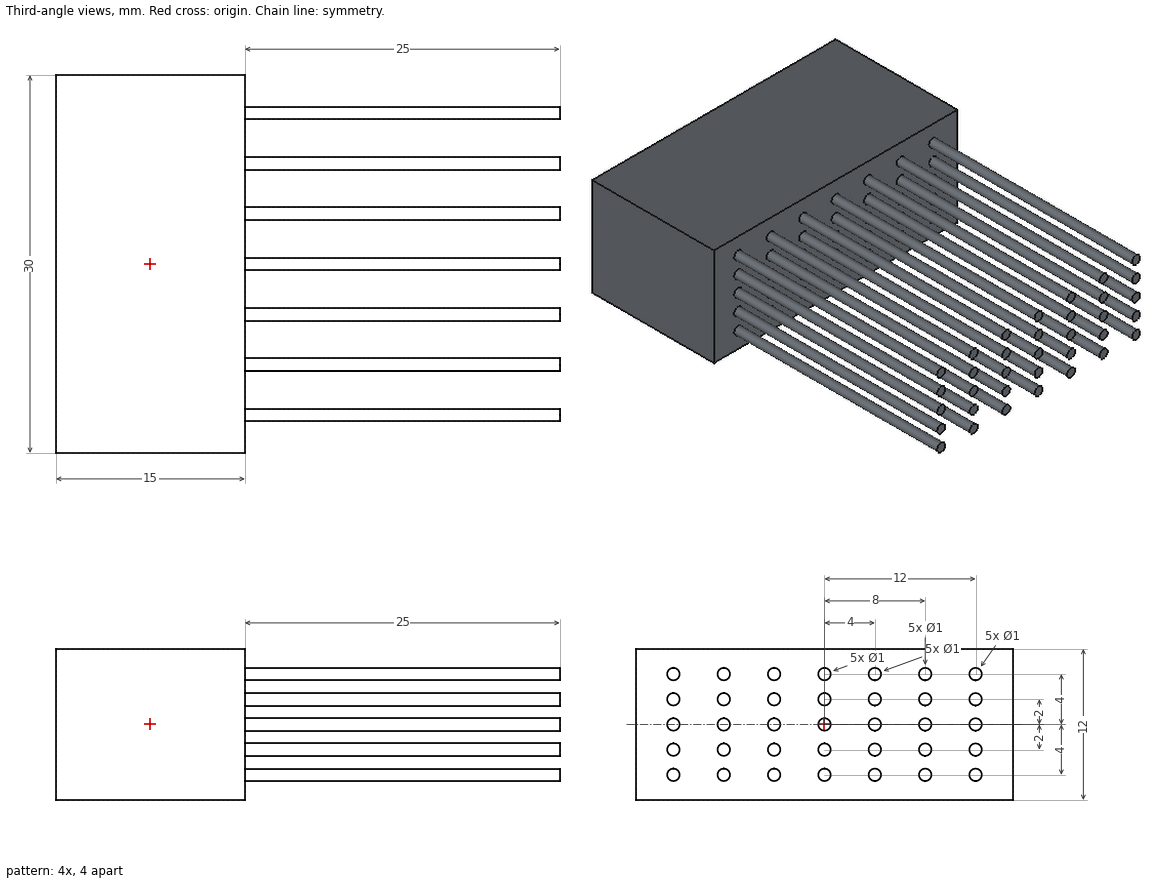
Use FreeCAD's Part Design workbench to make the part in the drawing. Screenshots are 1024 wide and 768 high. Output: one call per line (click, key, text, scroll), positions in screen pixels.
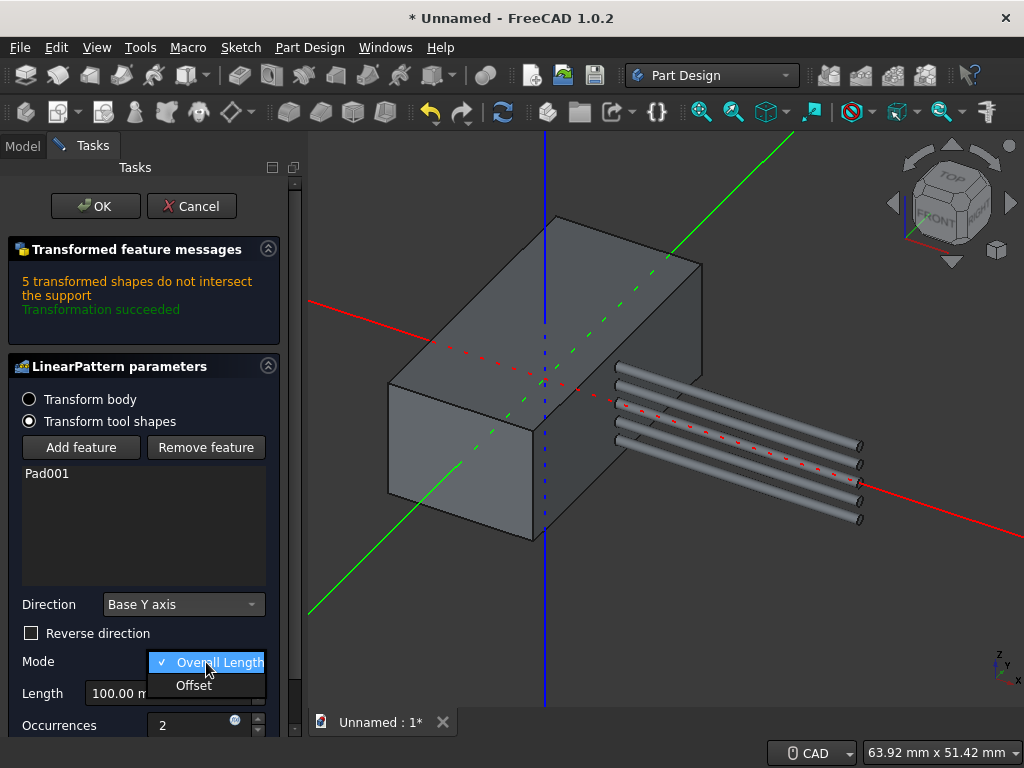
click(206, 686)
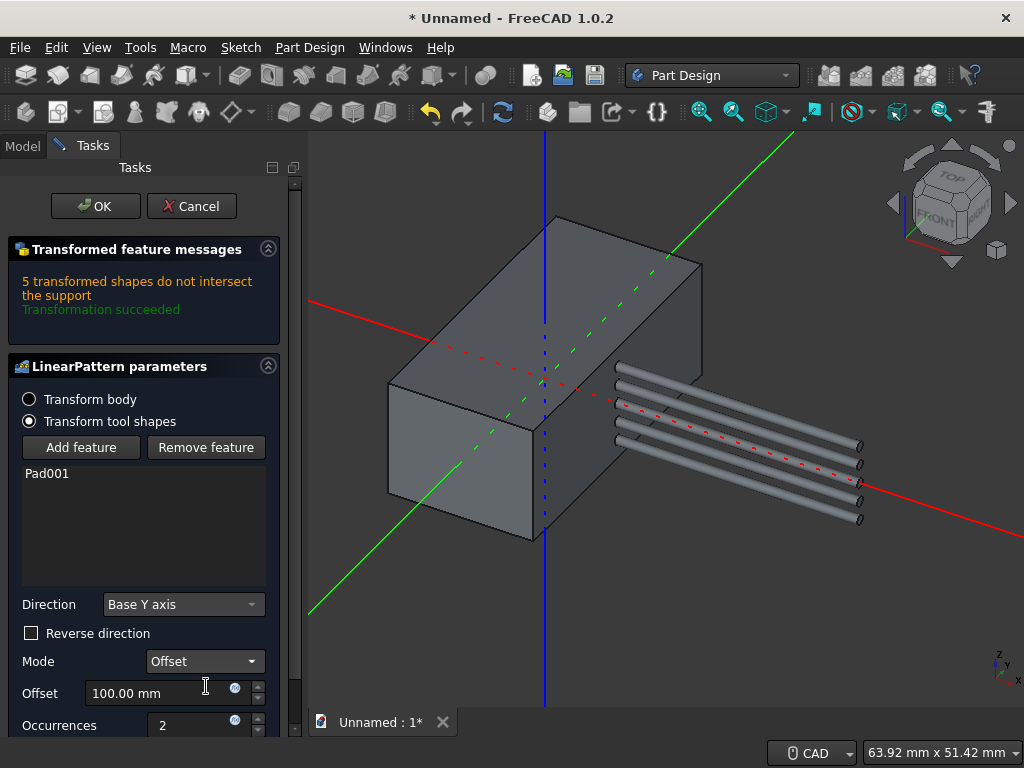
triple_click(168, 693)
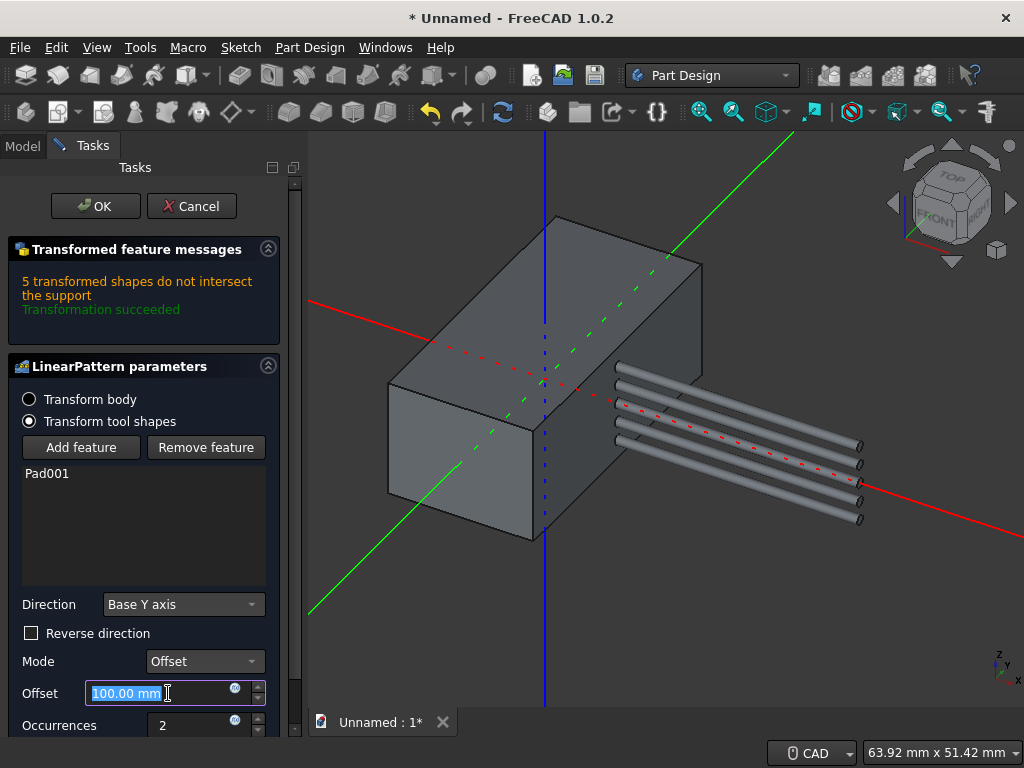
text(4)
key(Tab)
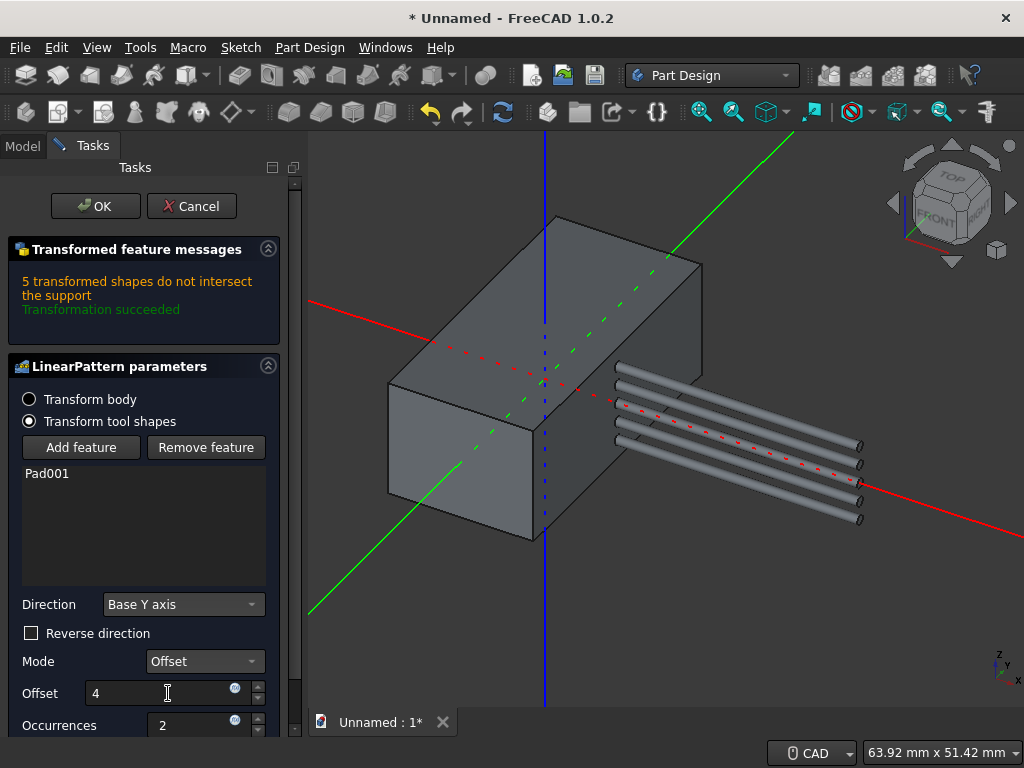
scroll(295, 456, down, 2)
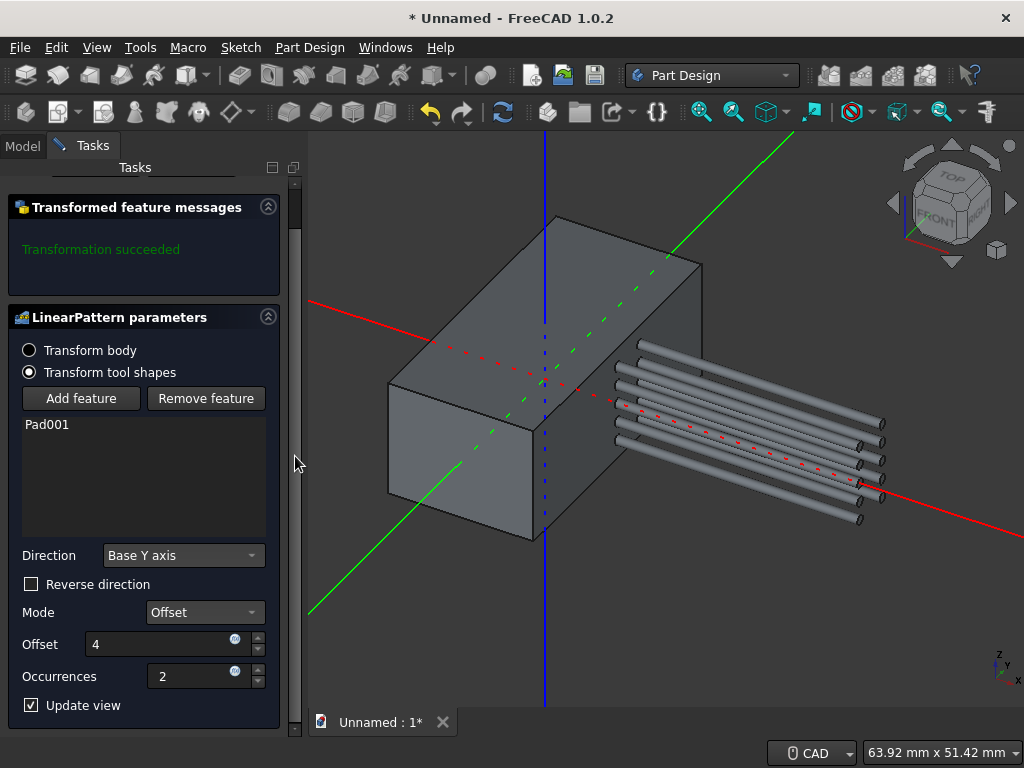
triple_click(198, 676)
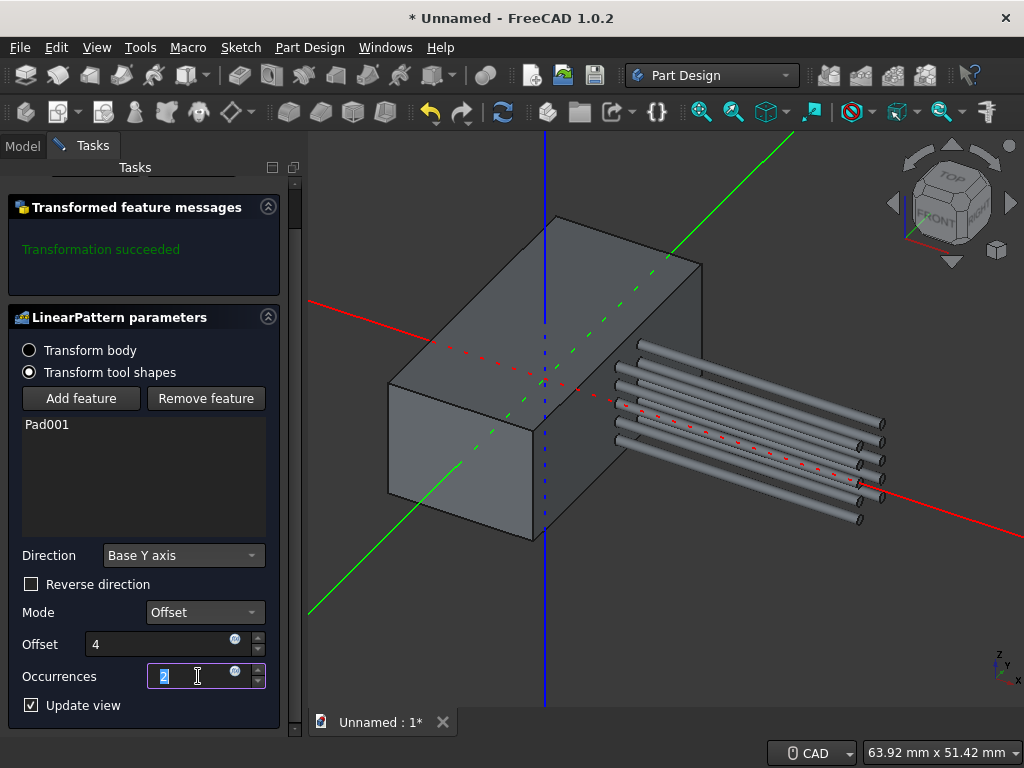
text(4)
key(Tab)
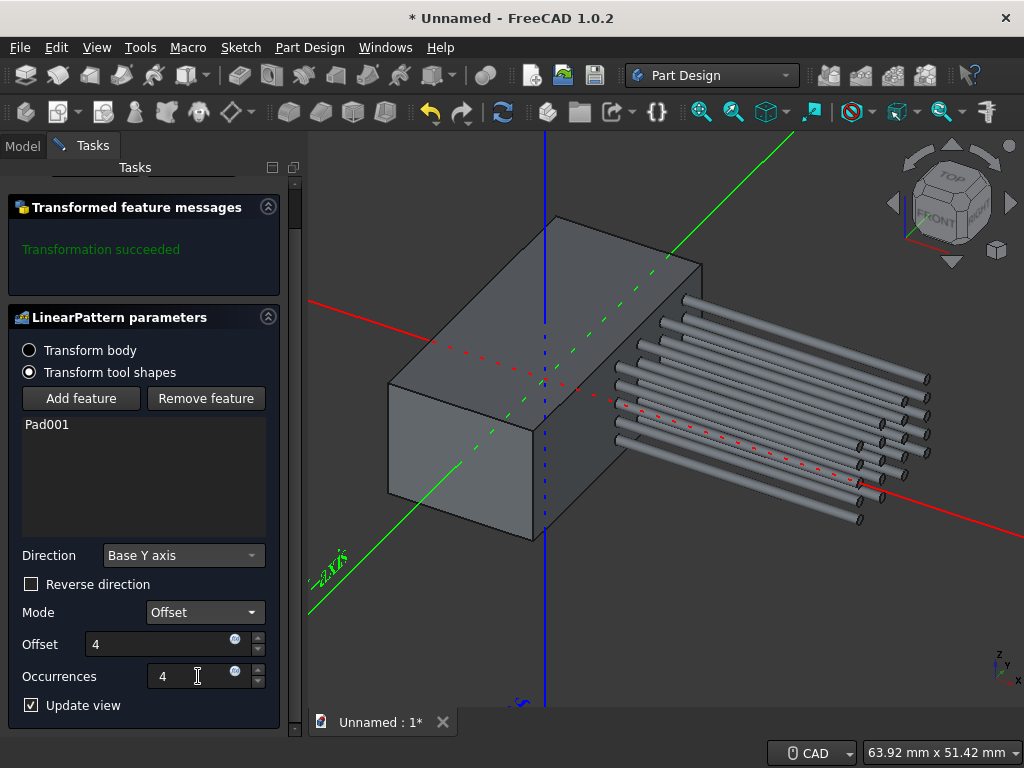
click(30, 584)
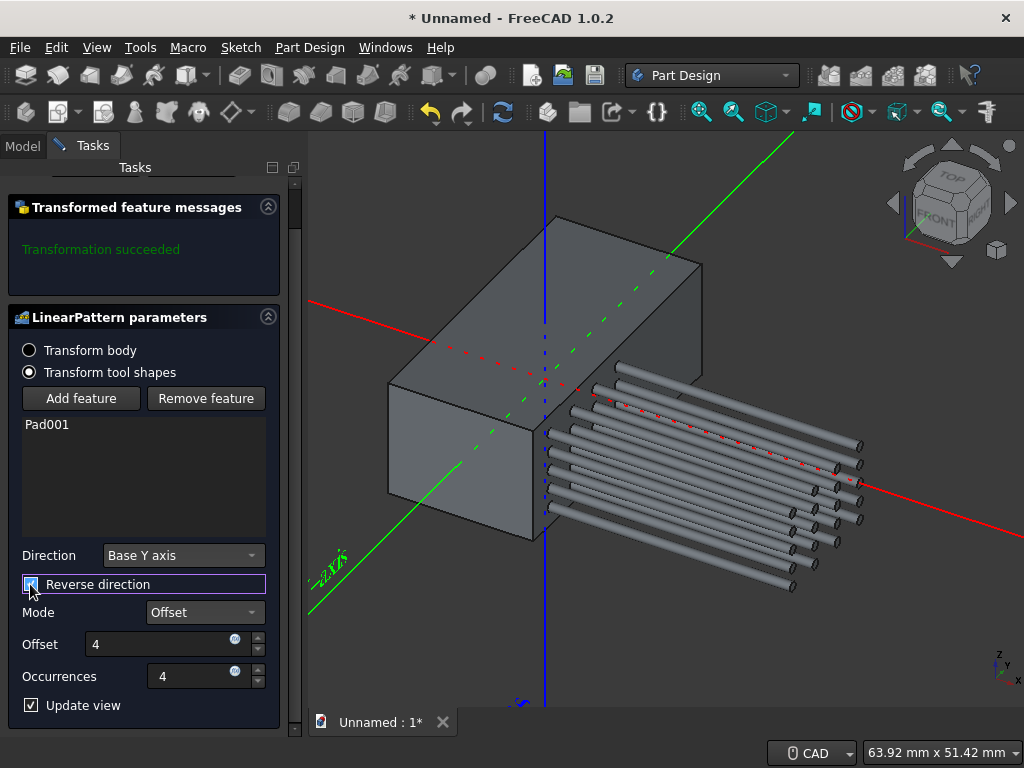
scroll(295, 456, up, 2)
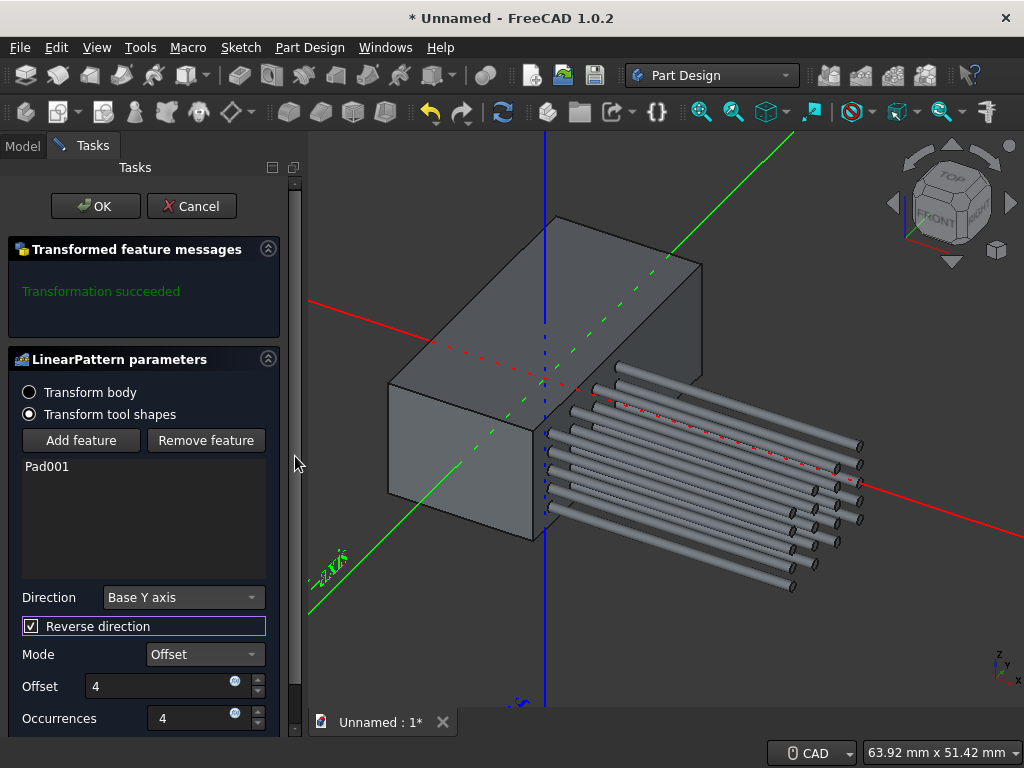
click(96, 206)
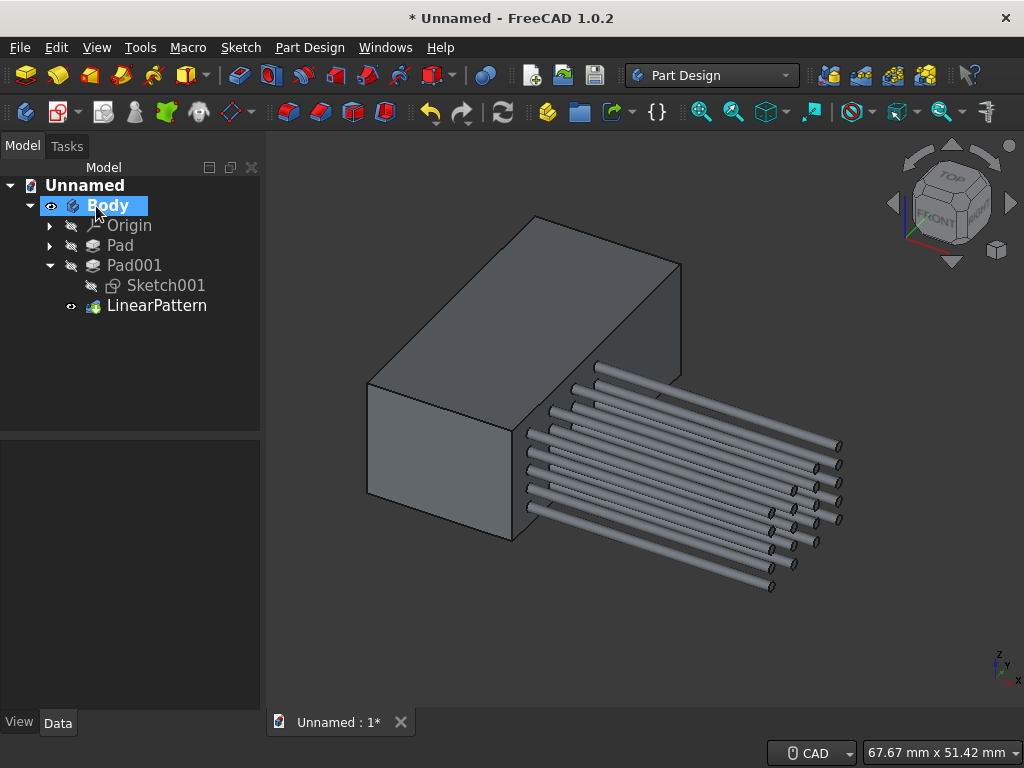
click(645, 354)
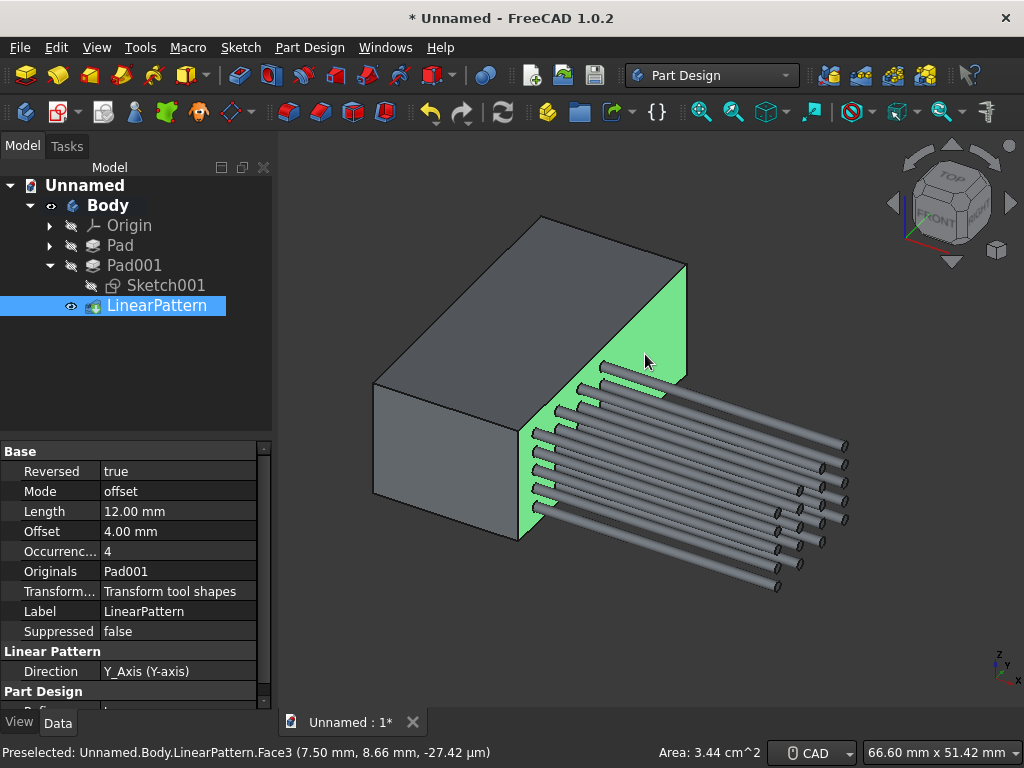
click(58, 112)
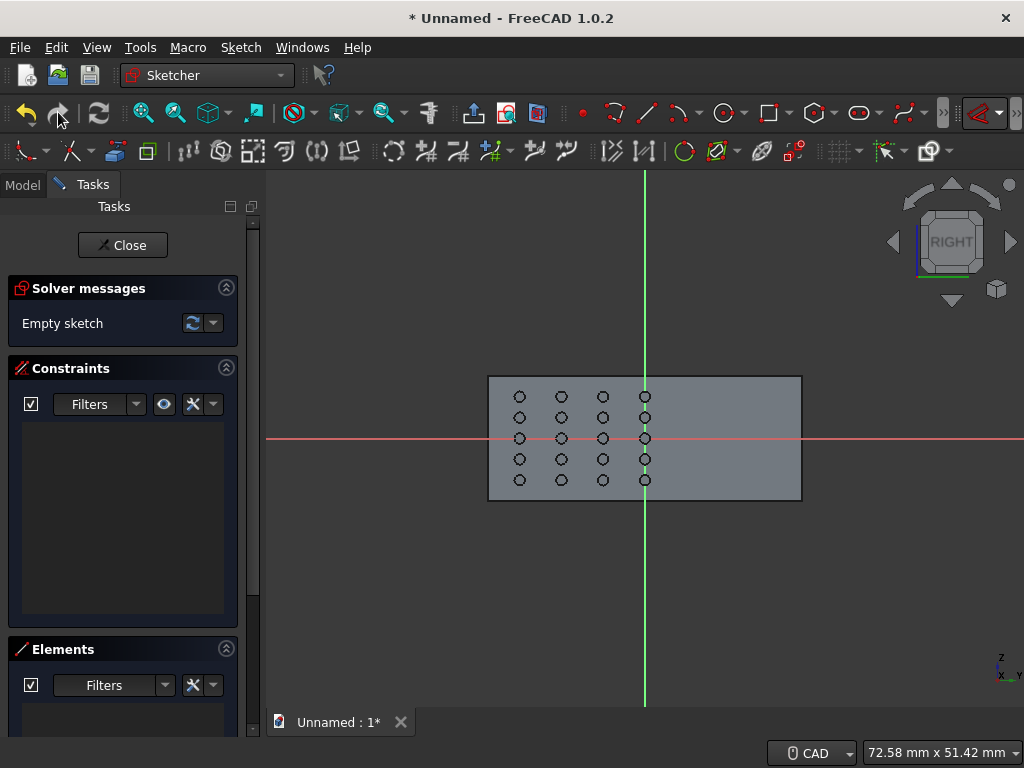
key(q)
key(s)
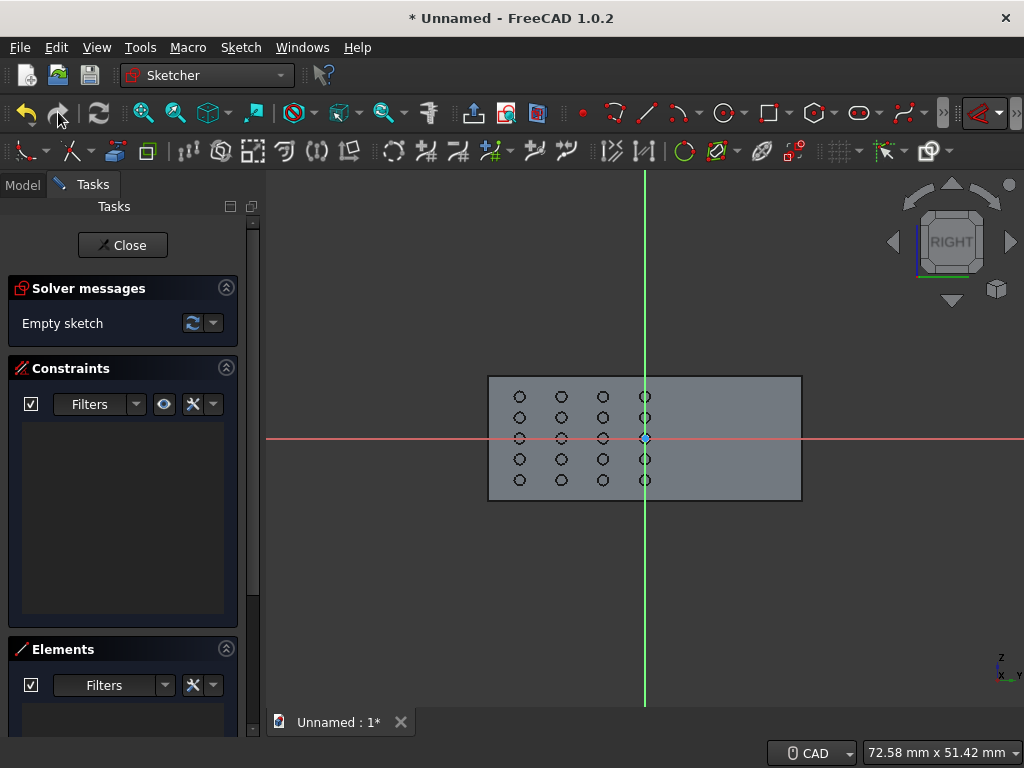
scroll(708, 438, up, 6)